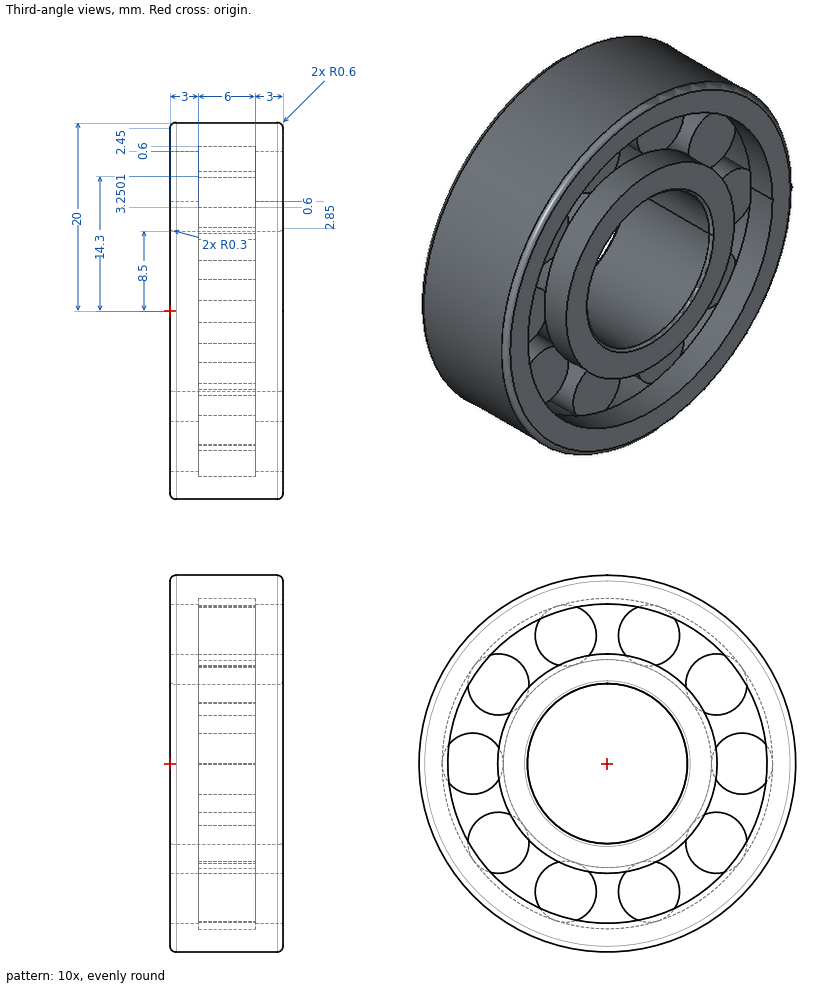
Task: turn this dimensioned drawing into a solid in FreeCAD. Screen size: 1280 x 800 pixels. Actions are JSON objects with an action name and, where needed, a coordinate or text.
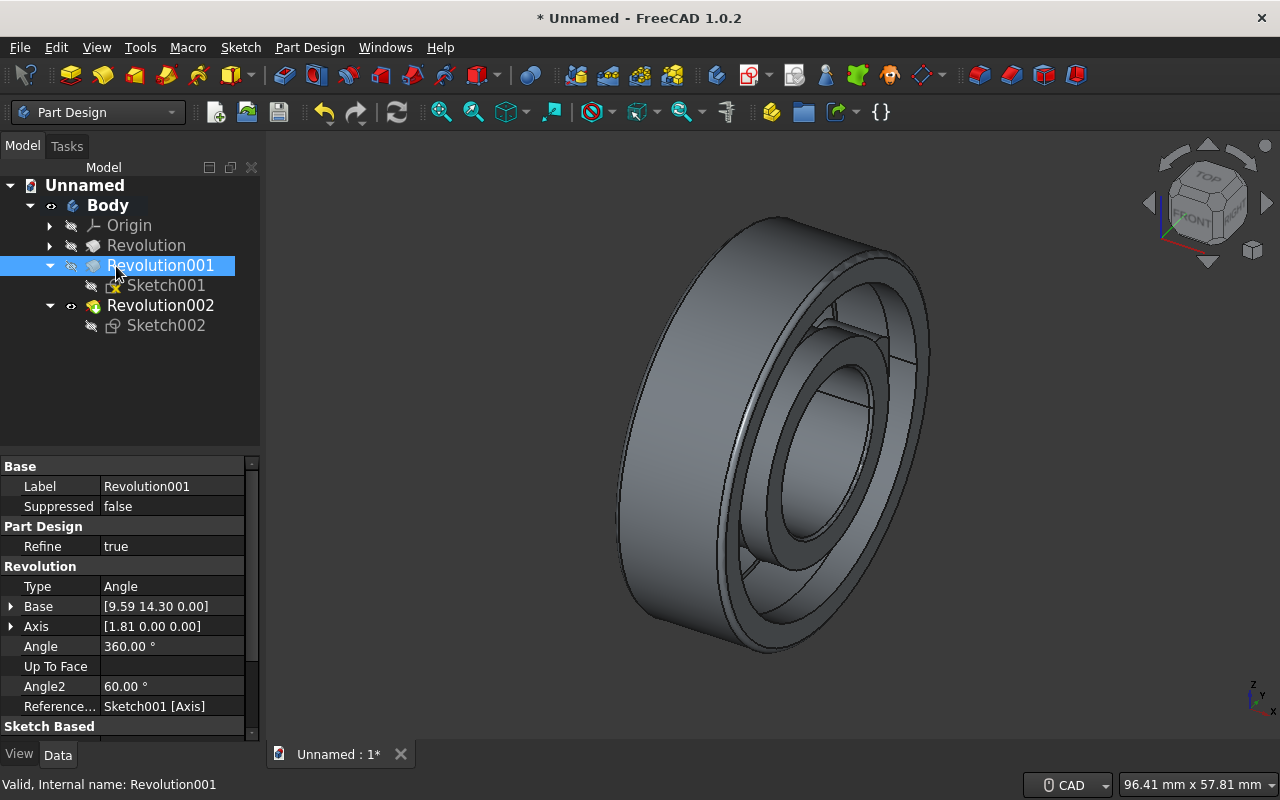
{"action": "left_click", "coordinate": [640, 76]}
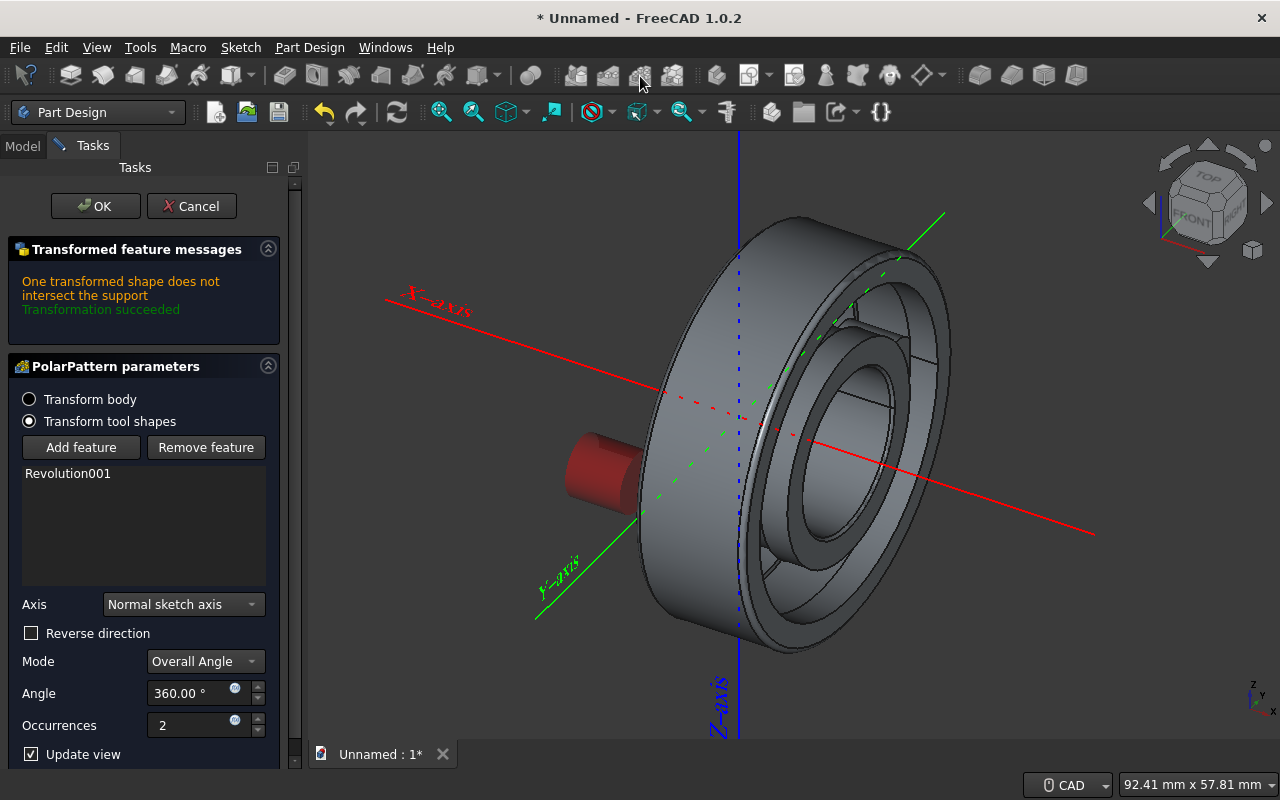
{"action": "left_click", "coordinate": [184, 604]}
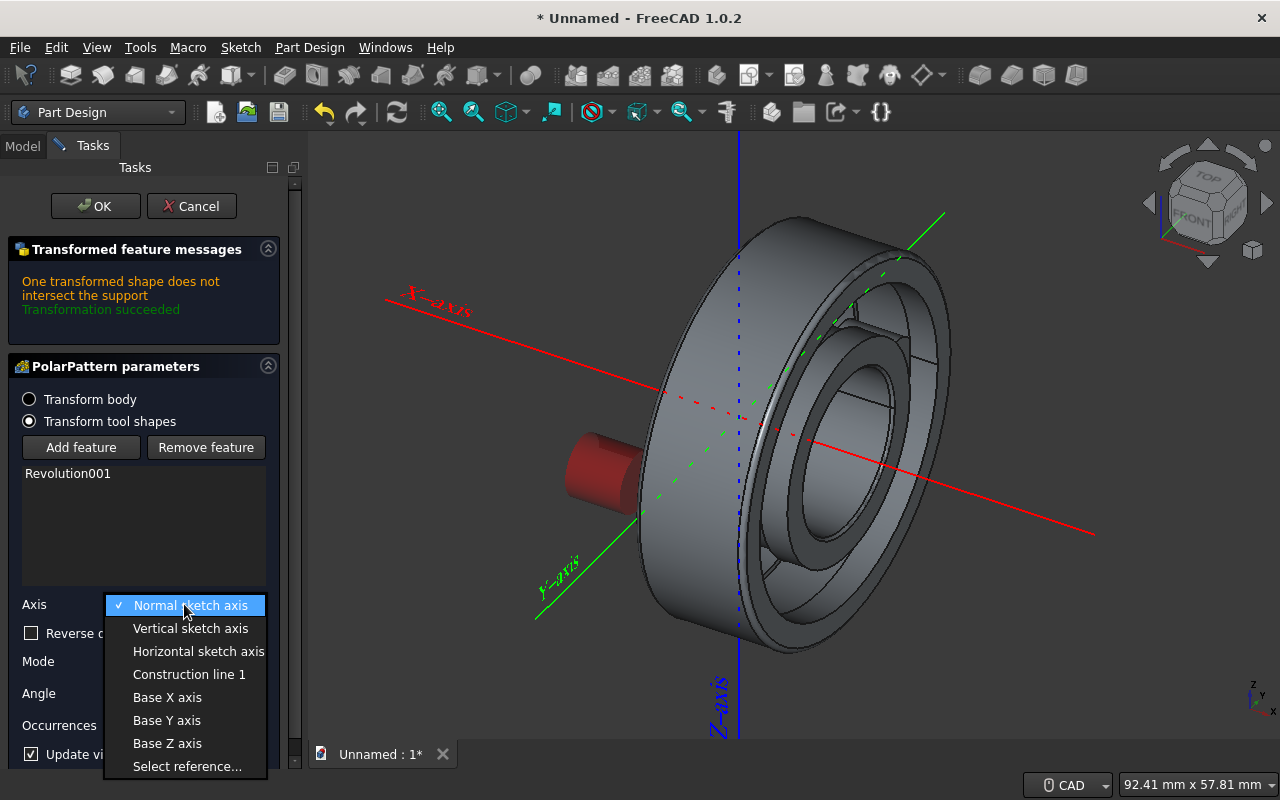
{"action": "left_click", "coordinate": [184, 698]}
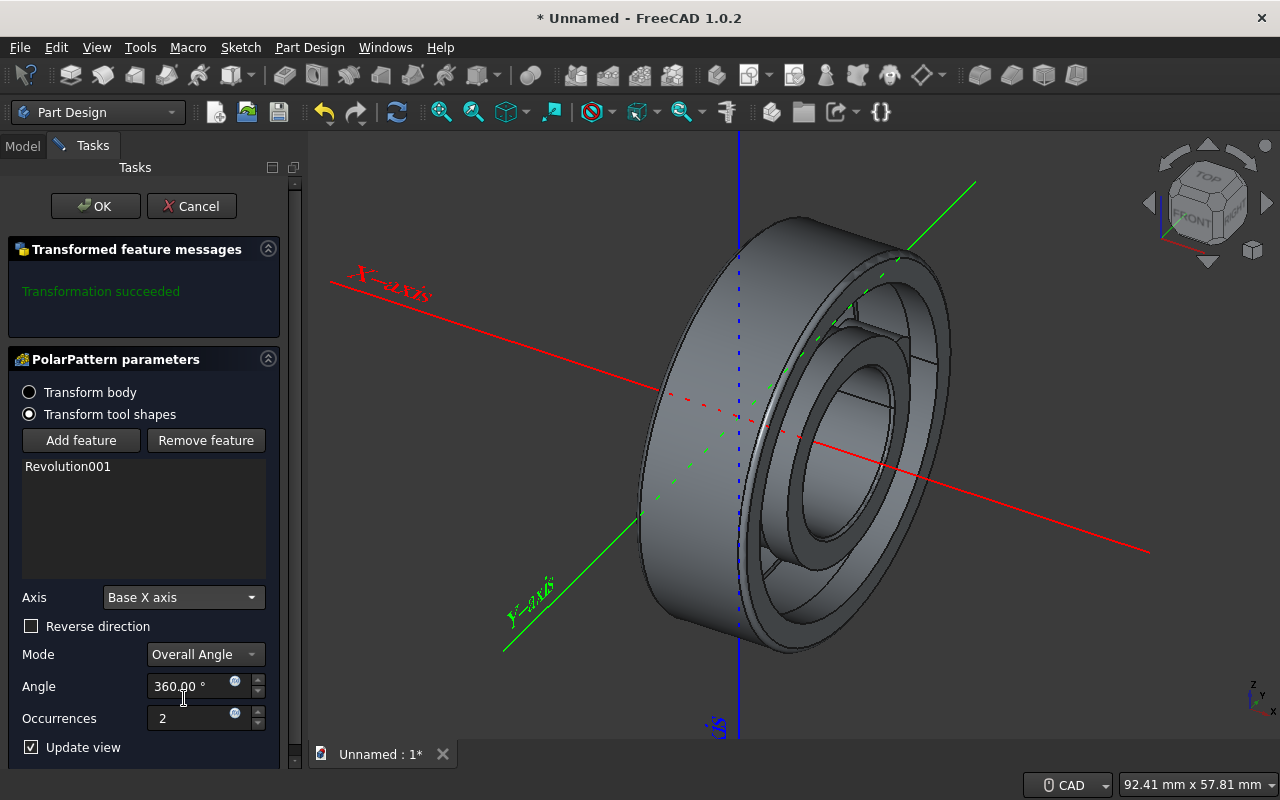
{"action": "triple_click", "coordinate": [198, 718]}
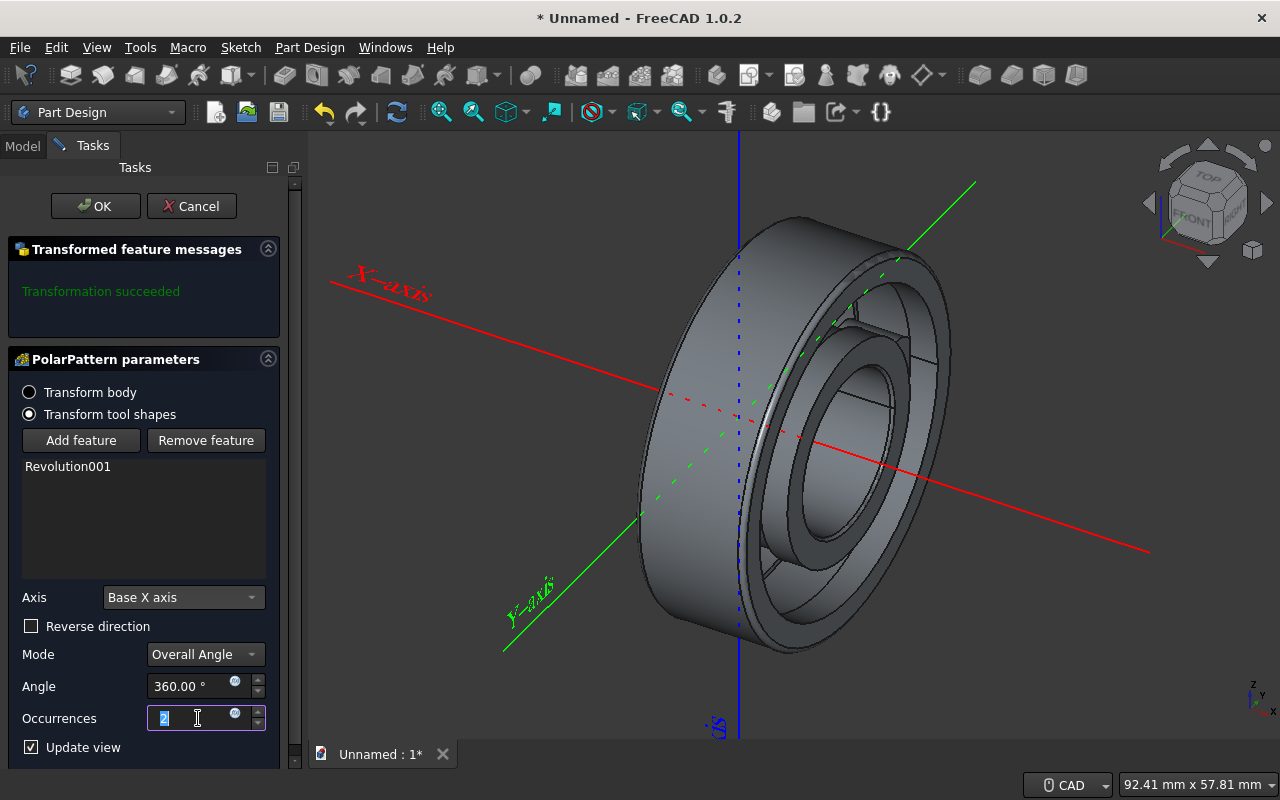
{"action": "type", "text": "10"}
{"action": "key", "text": "Tab"}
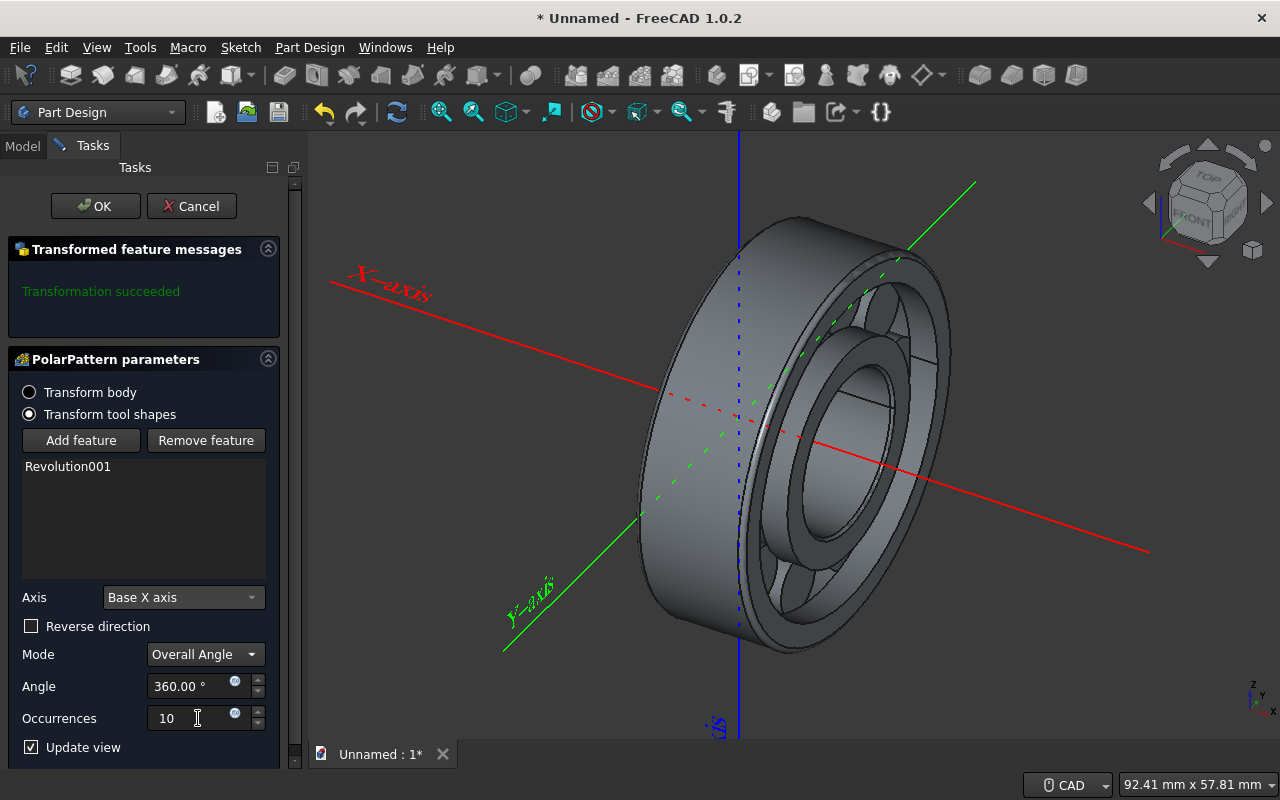
{"action": "left_click", "coordinate": [96, 206]}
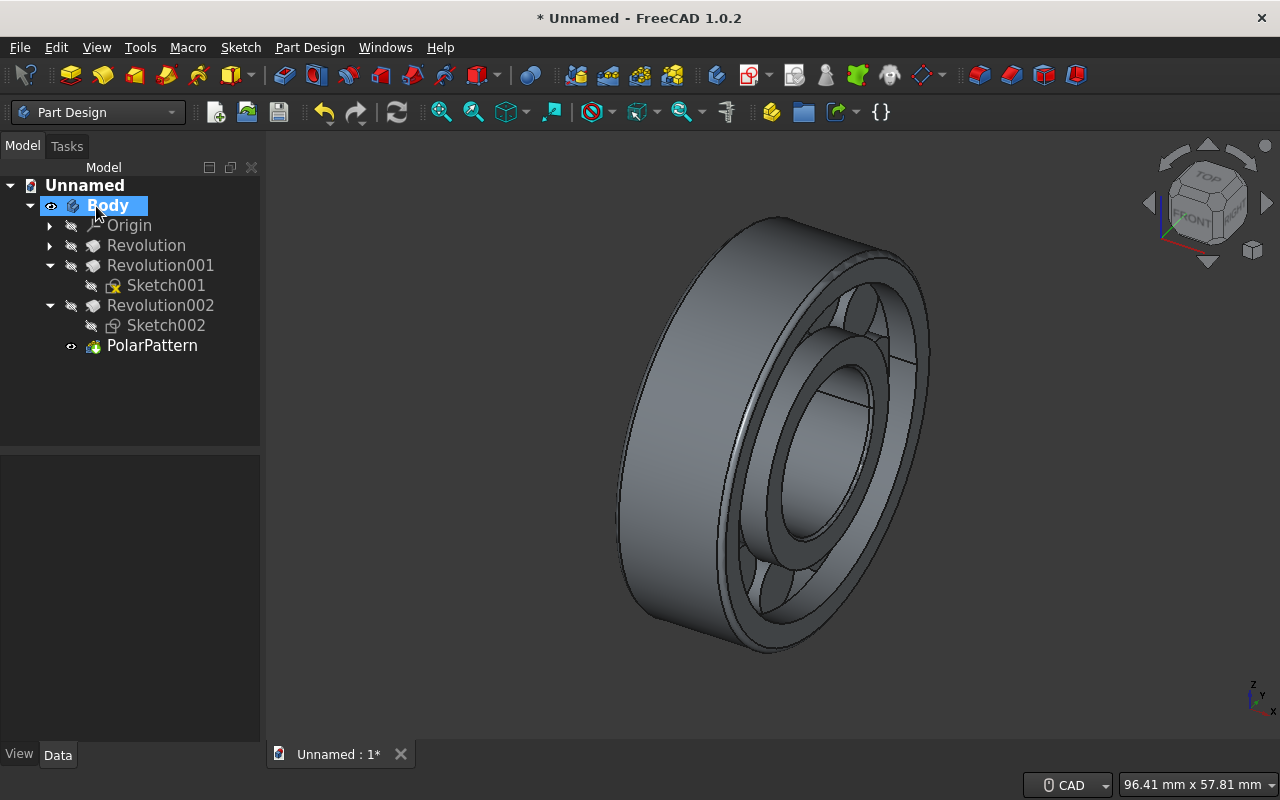
{"action": "key", "text": "0"}